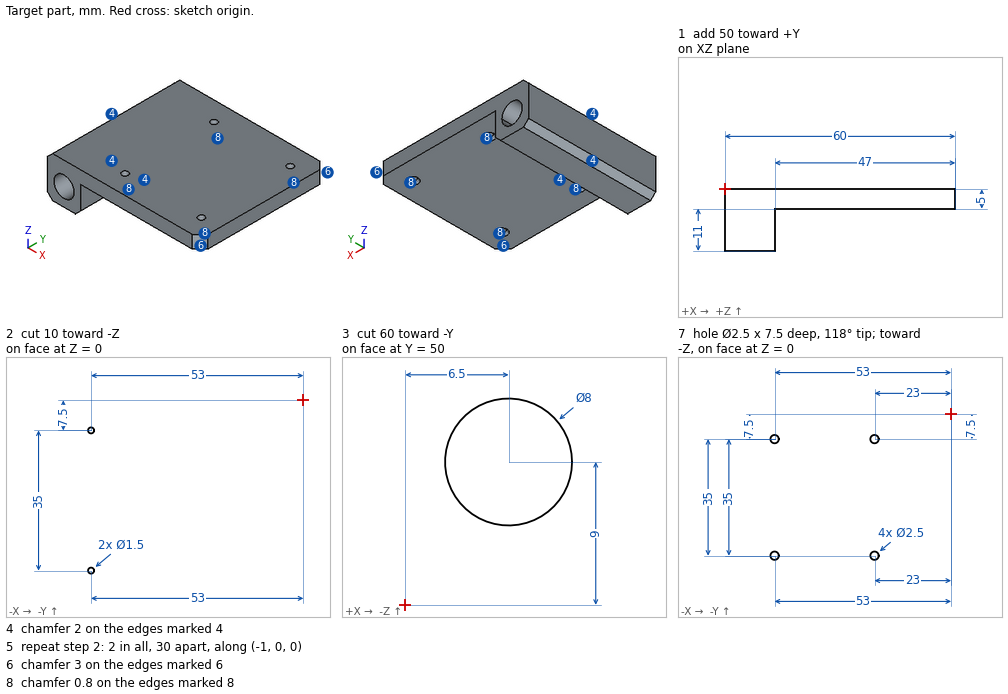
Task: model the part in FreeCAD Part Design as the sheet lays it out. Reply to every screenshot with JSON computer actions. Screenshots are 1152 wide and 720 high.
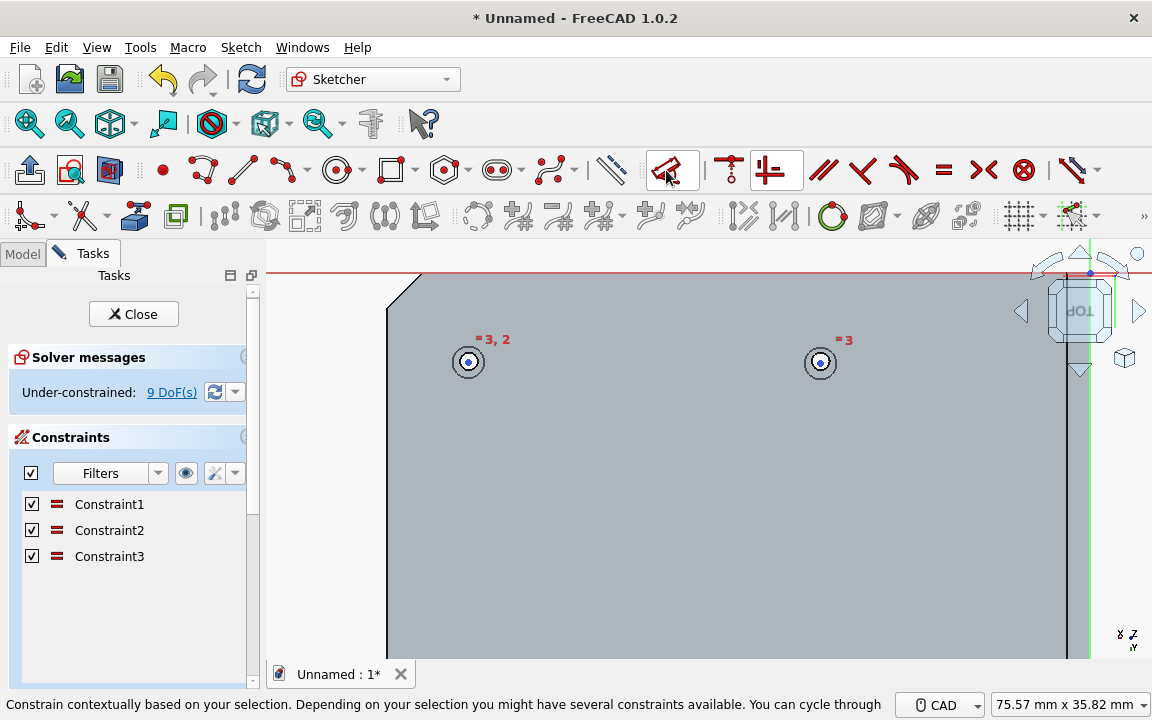
{"action": "scroll", "coordinate": [480, 351], "scroll_direction": "down", "scroll_amount": 3}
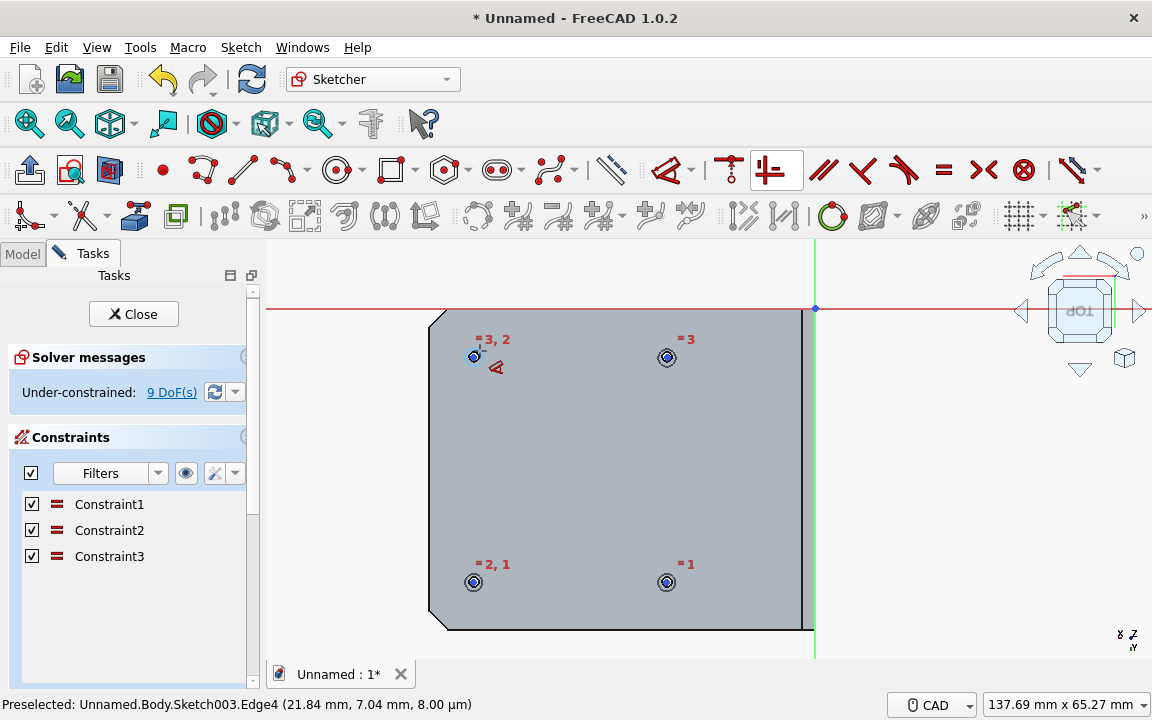
{"action": "scroll", "coordinate": [673, 576], "scroll_direction": "up", "scroll_amount": 5}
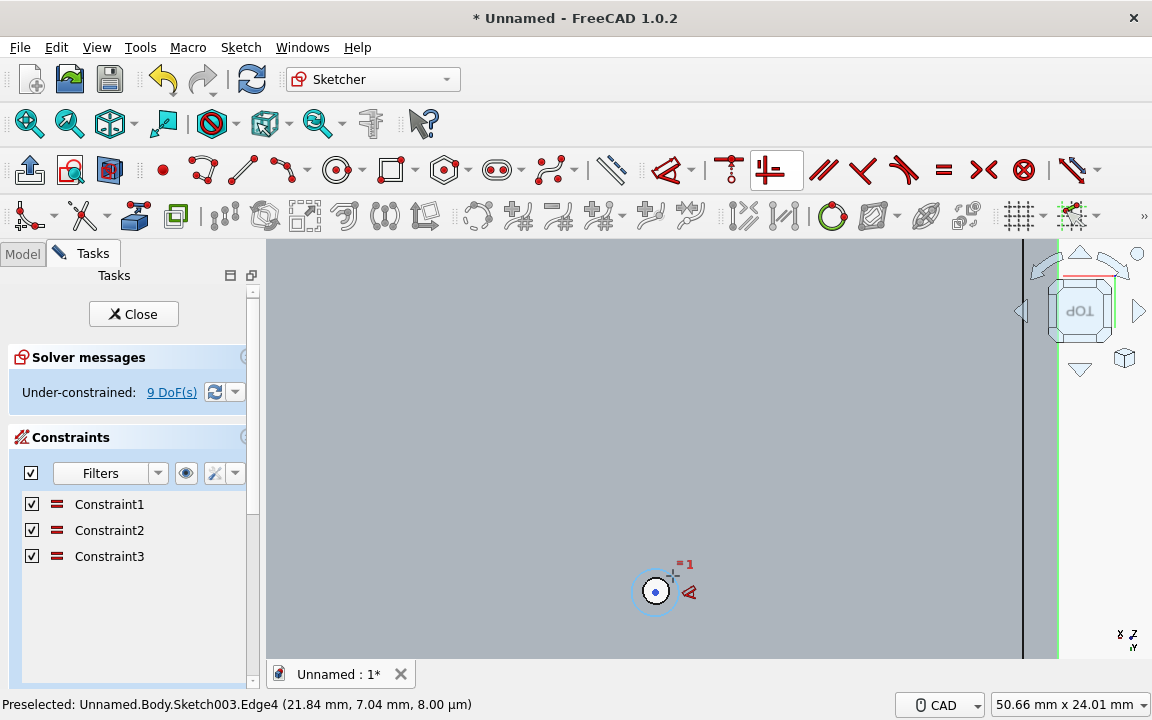
{"action": "left_click", "coordinate": [672, 576]}
{"action": "left_click", "coordinate": [695, 554]}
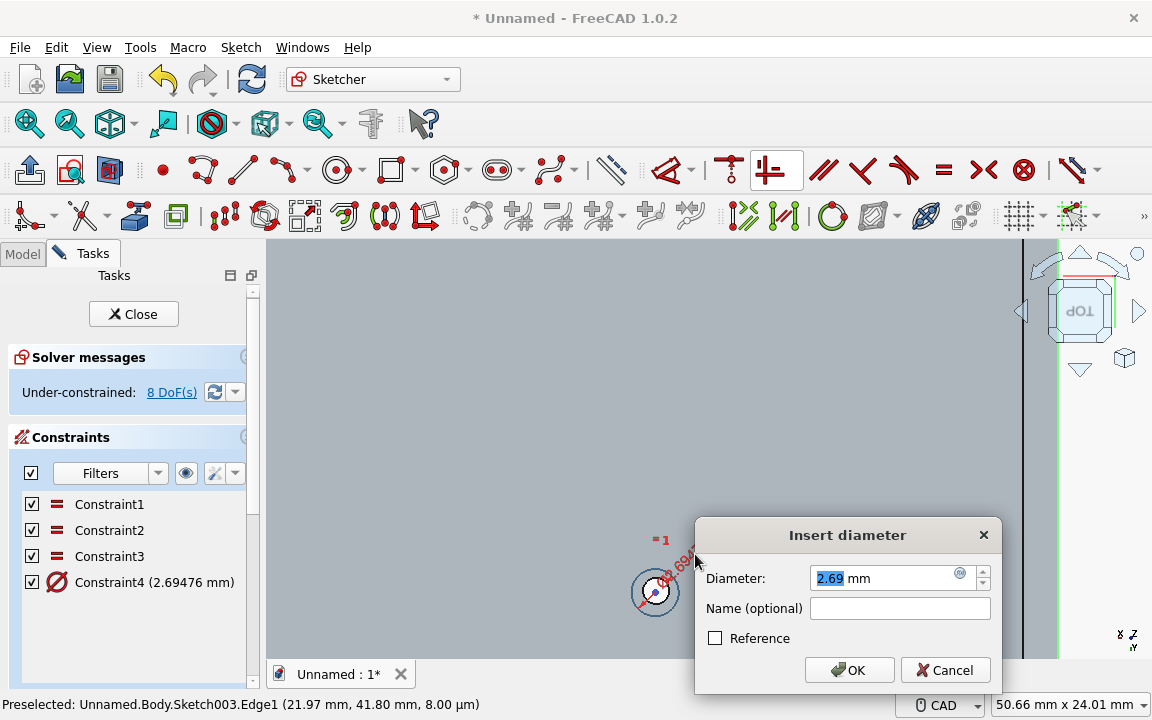
{"action": "type", "text": "2.5"}
{"action": "key", "text": "Return"}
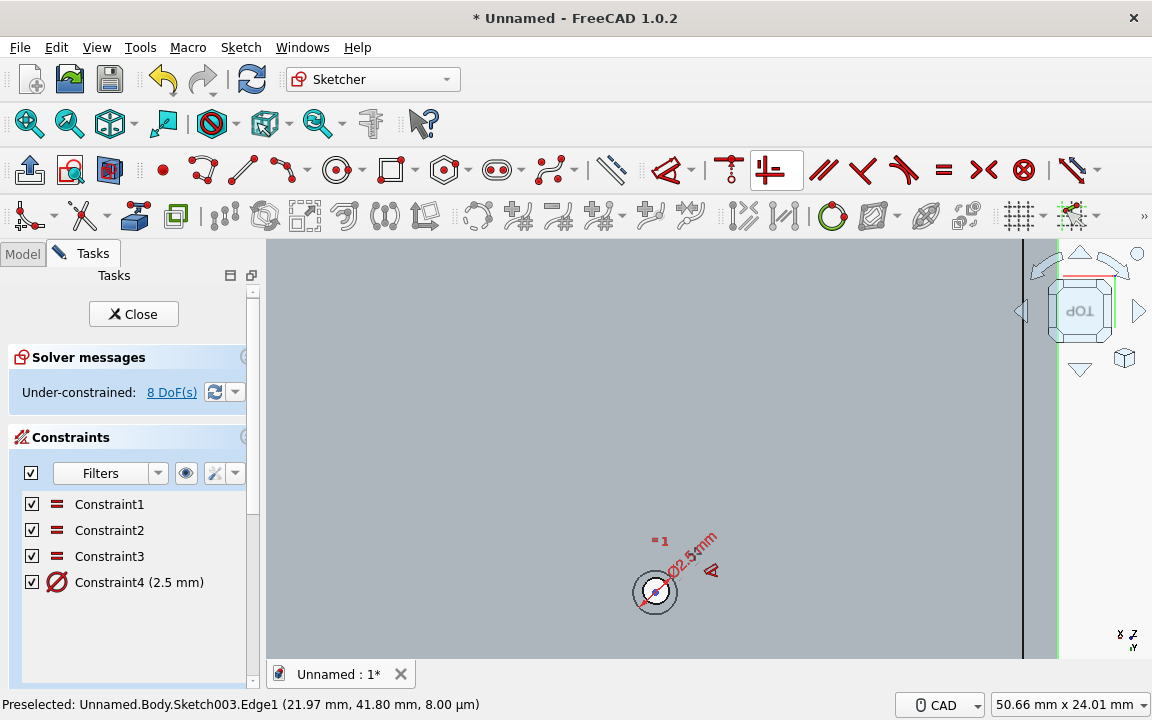
{"action": "left_click", "coordinate": [655, 593]}
{"action": "left_click", "coordinate": [821, 627]}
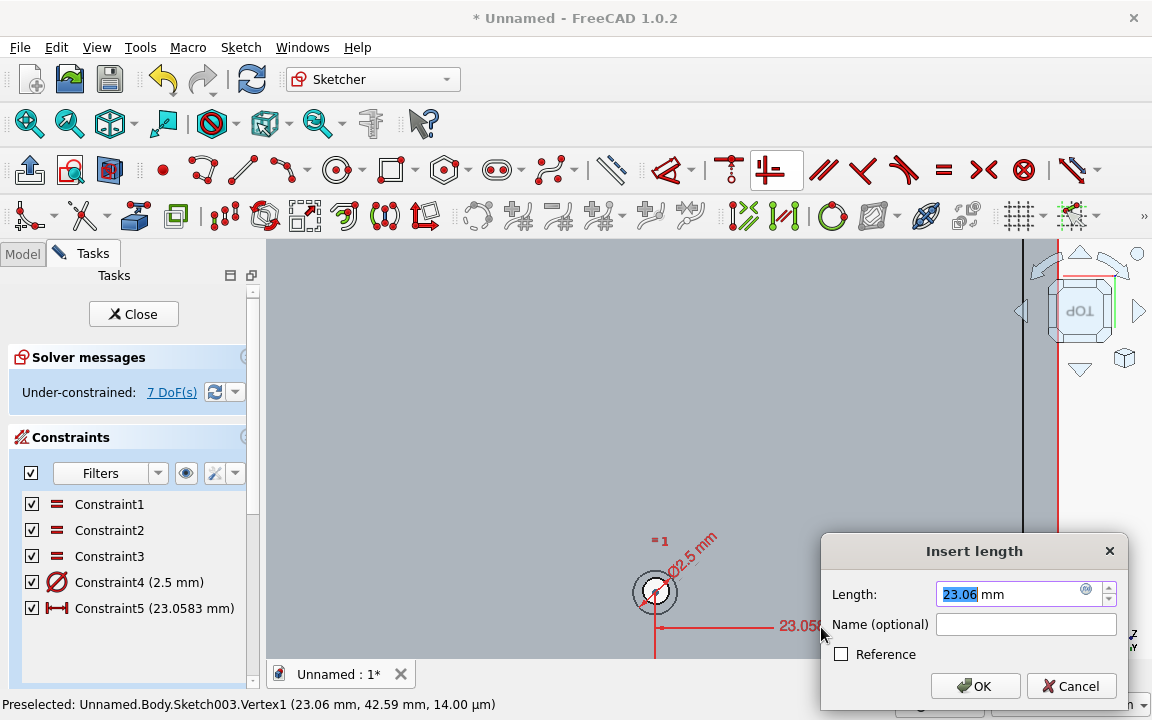
{"action": "type", "text": "23"}
{"action": "key", "text": "Return"}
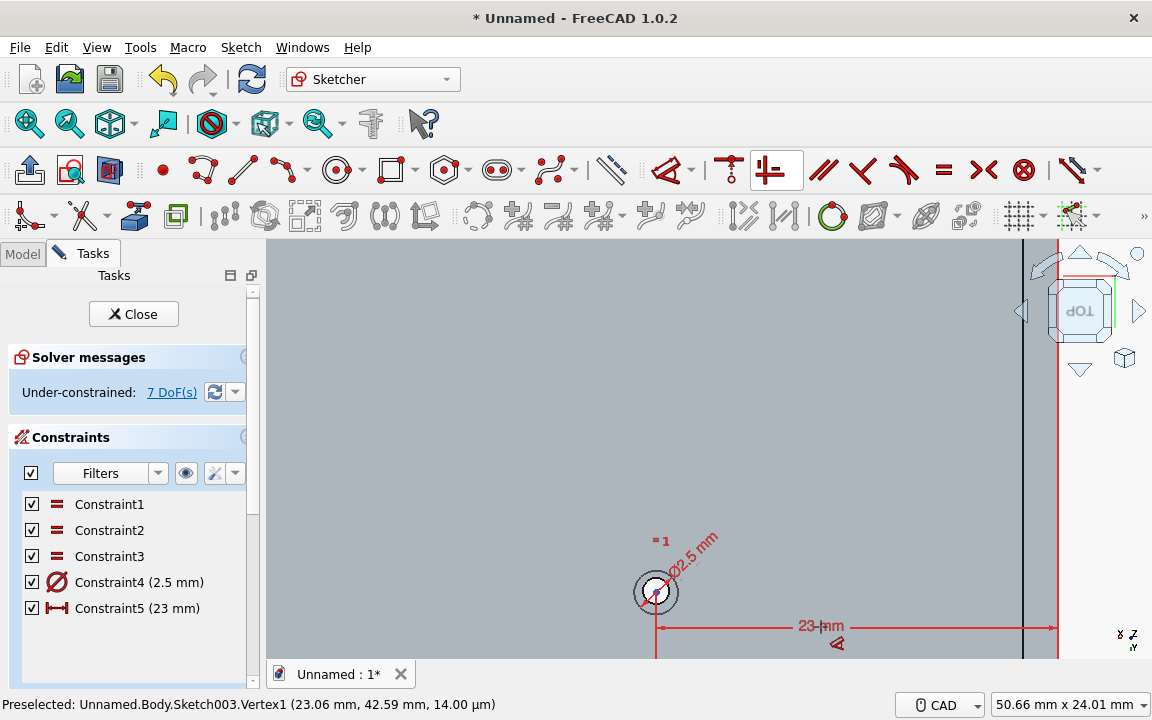
{"action": "scroll", "coordinate": [673, 576], "scroll_direction": "down", "scroll_amount": 5}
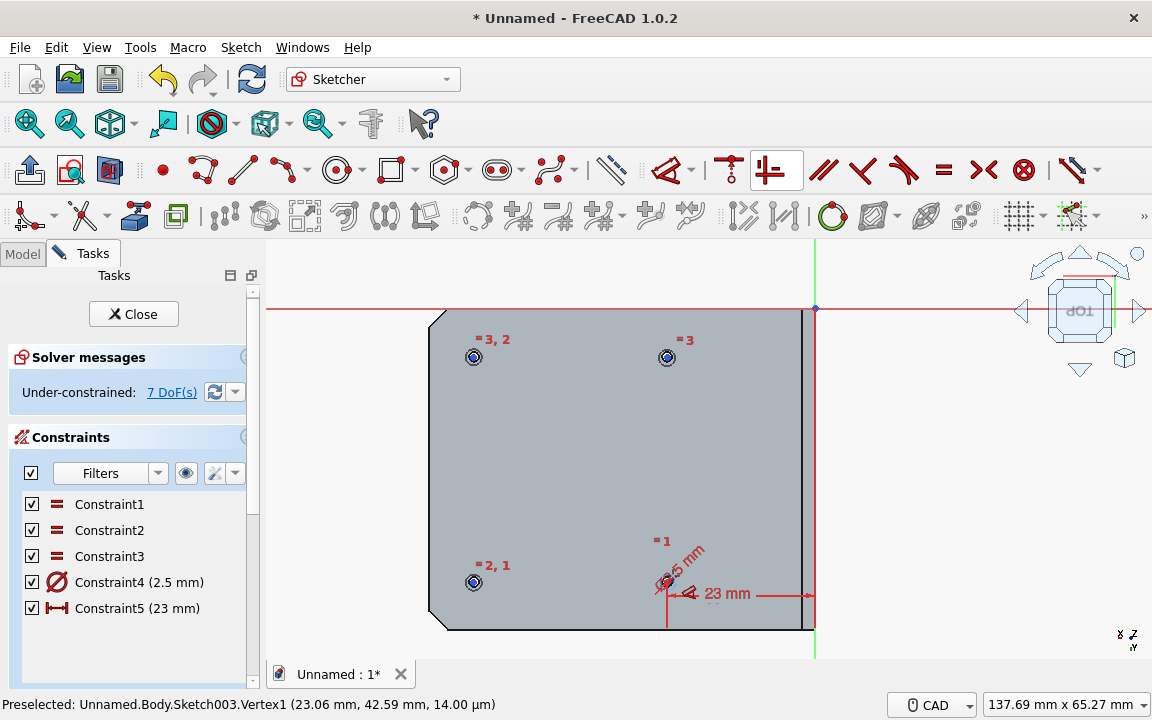
{"action": "left_click", "coordinate": [474, 583]}
{"action": "left_click", "coordinate": [644, 275]}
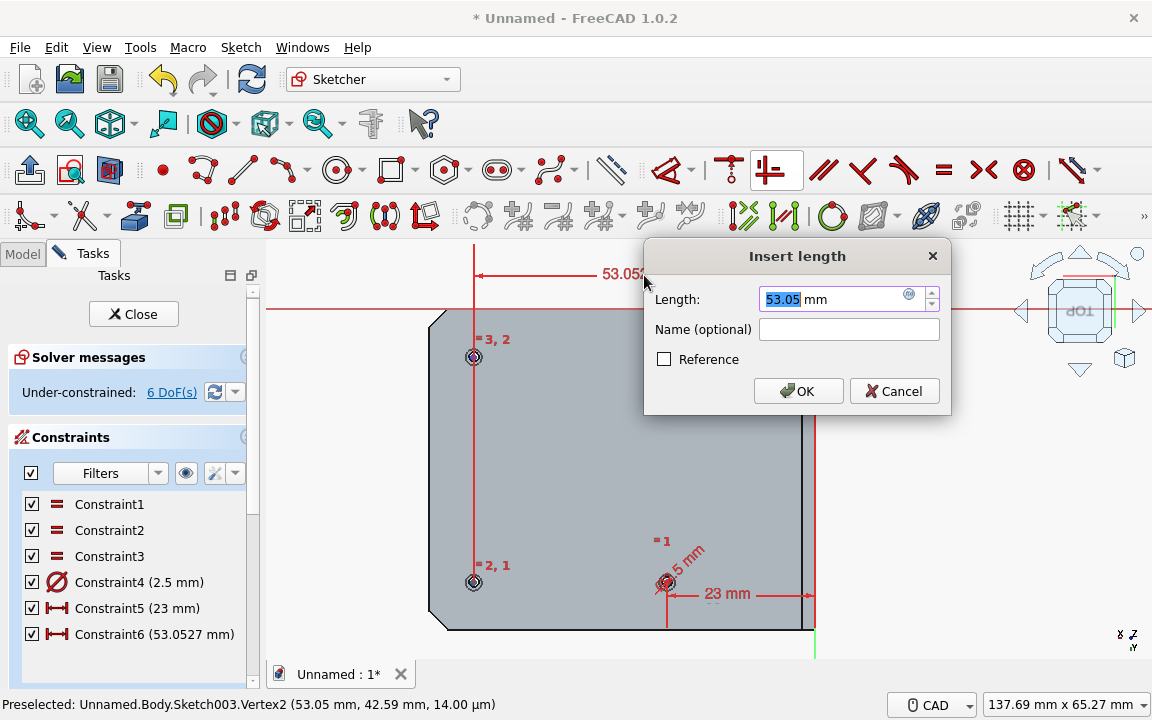
{"action": "type", "text": "53"}
{"action": "key", "text": "Return"}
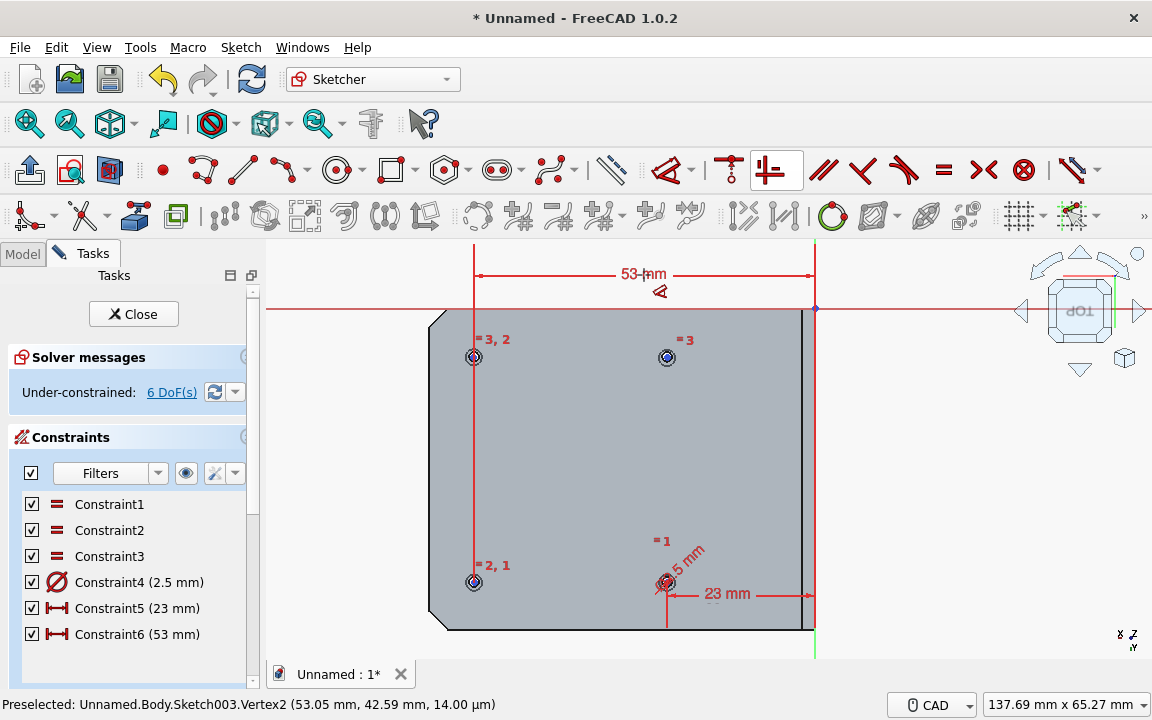
{"action": "left_click", "coordinate": [474, 357]}
{"action": "left_click", "coordinate": [566, 275]}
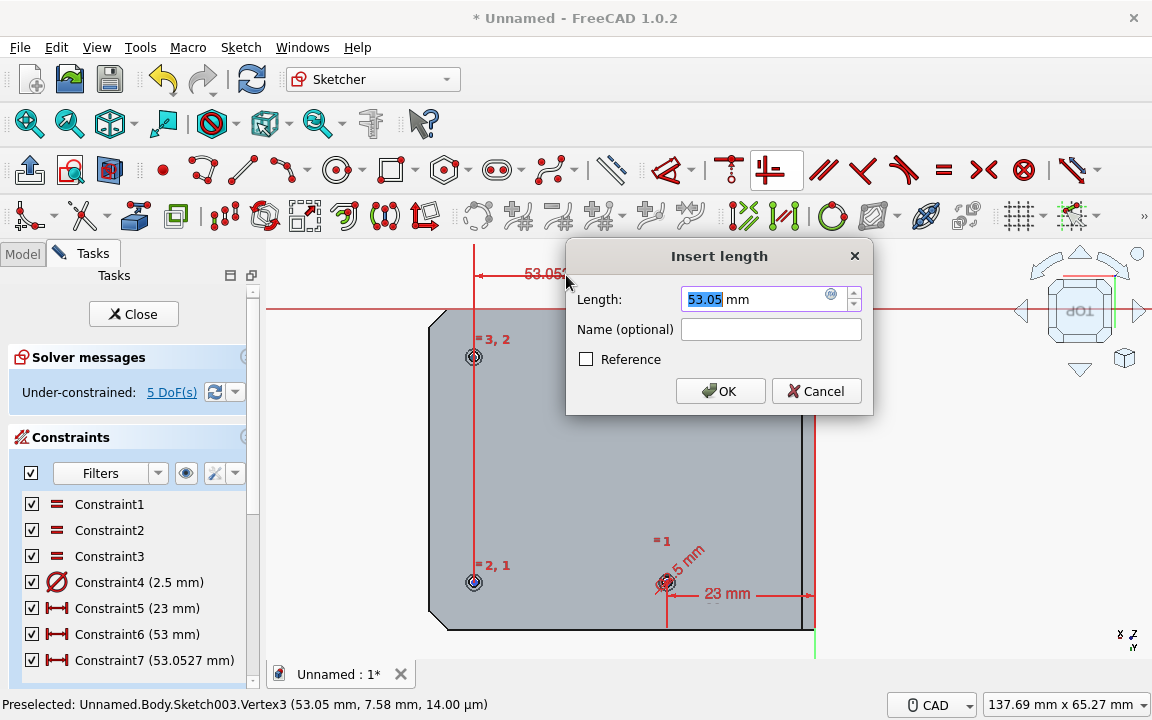
{"action": "type", "text": "53"}
{"action": "key", "text": "Return"}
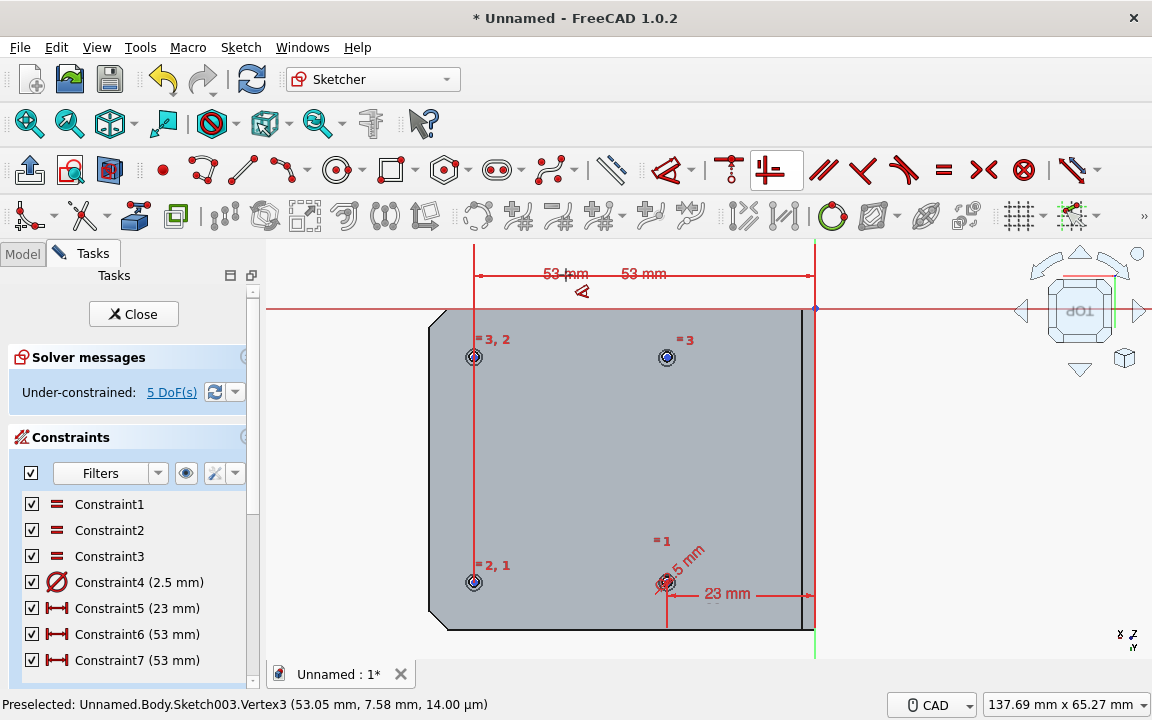
{"action": "left_click", "coordinate": [667, 358]}
{"action": "left_click", "coordinate": [741, 275]}